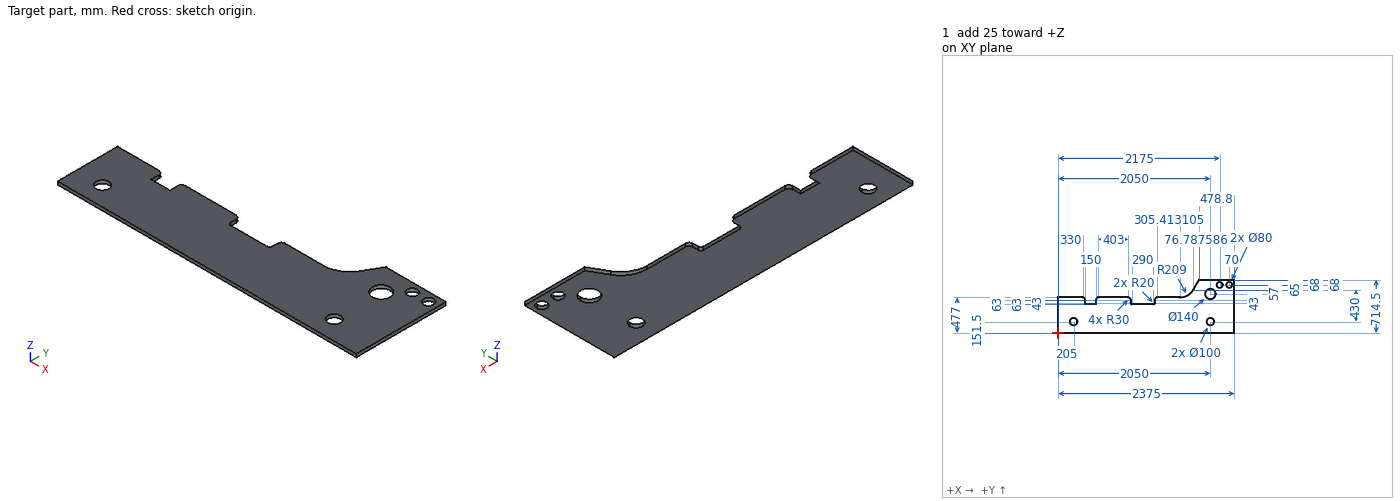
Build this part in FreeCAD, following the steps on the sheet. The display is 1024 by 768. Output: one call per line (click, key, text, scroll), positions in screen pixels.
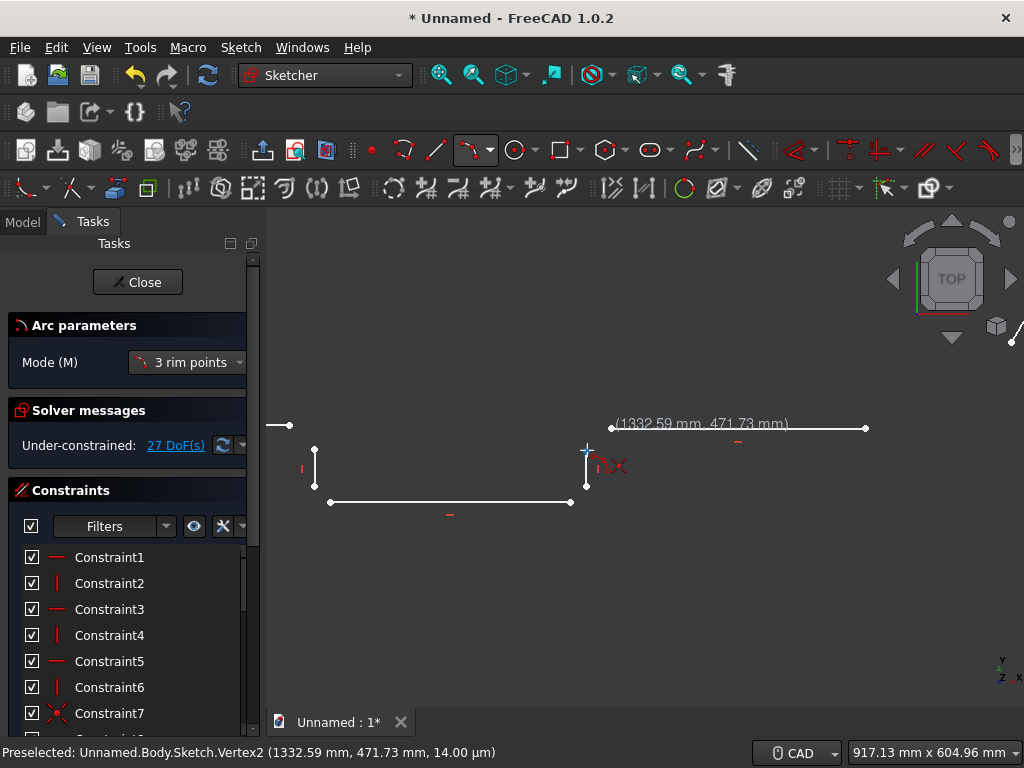
click(586, 452)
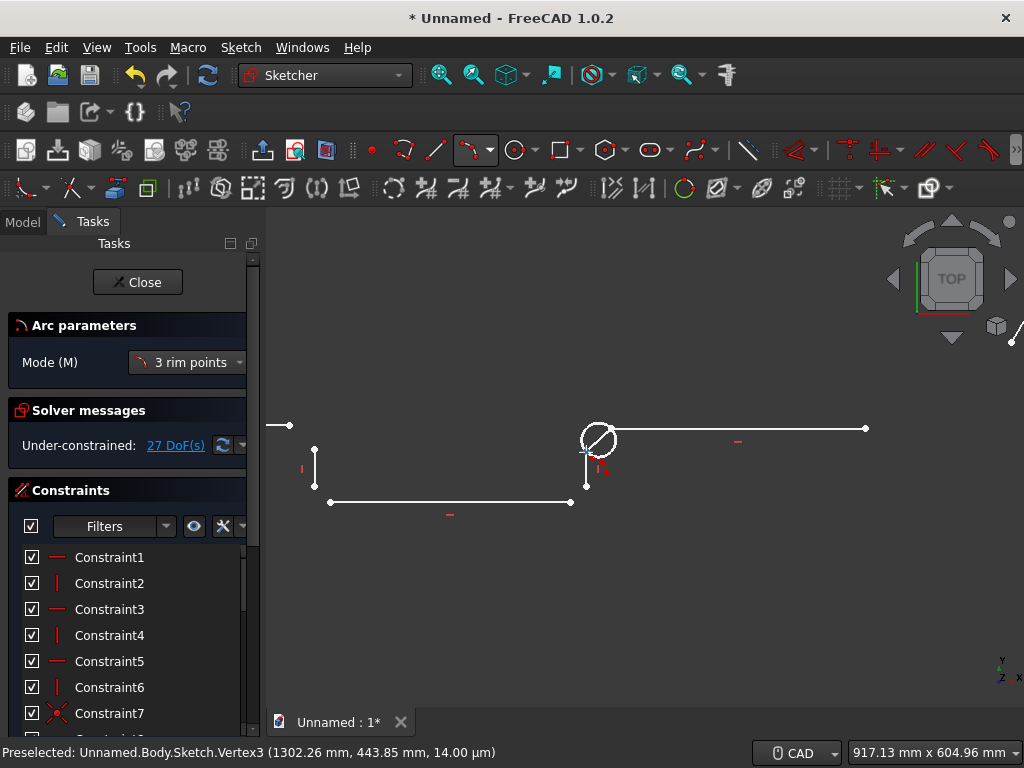
scroll(594, 431, up, 4)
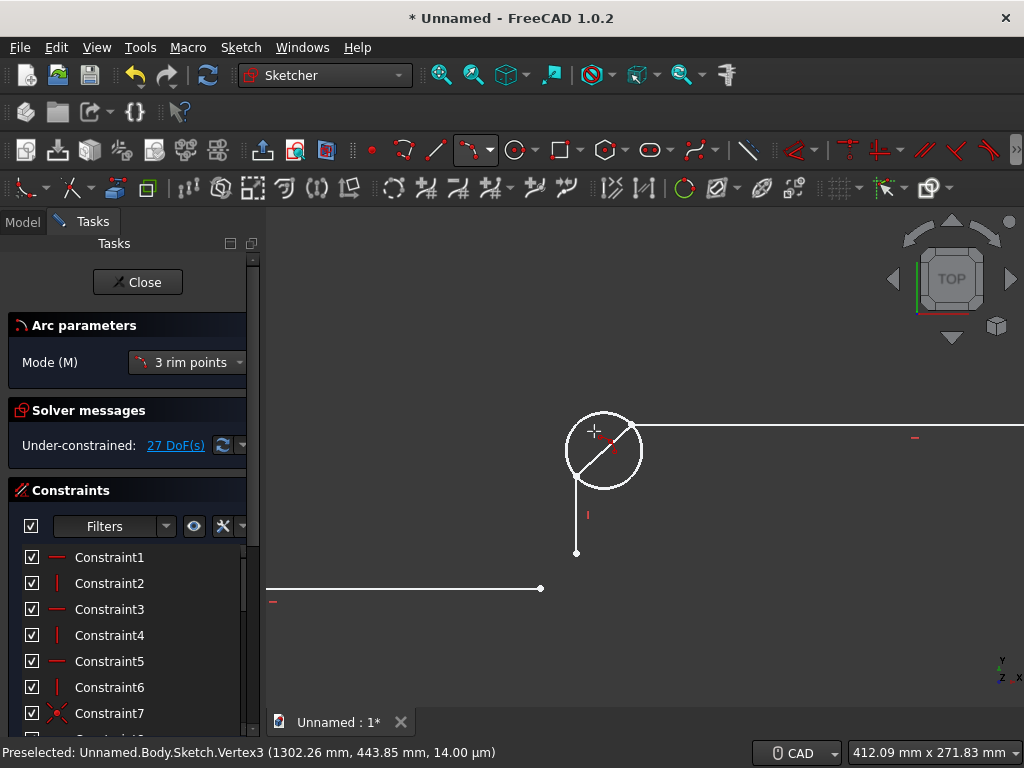
click(594, 431)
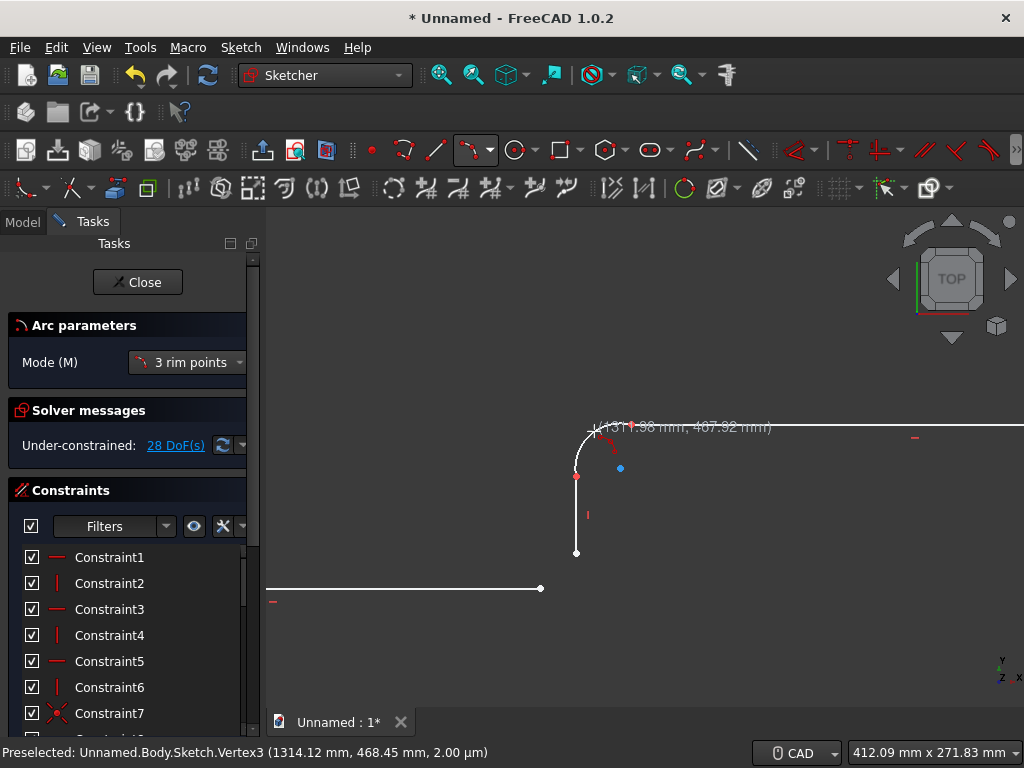
click(576, 553)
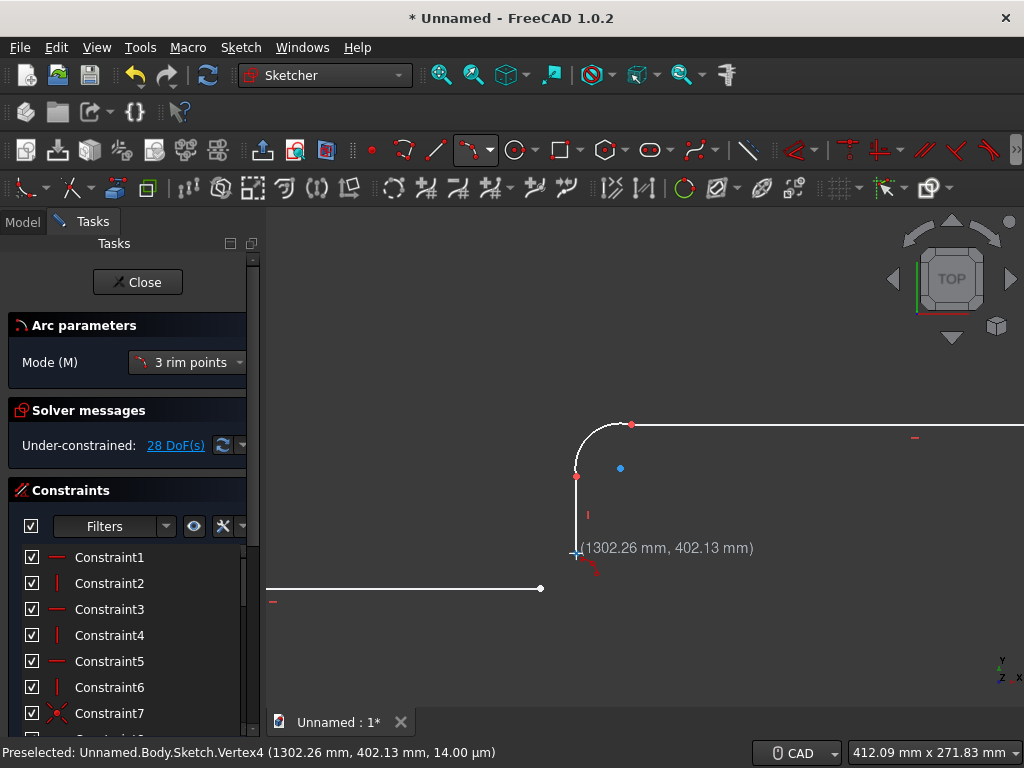
scroll(598, 439, down, 12)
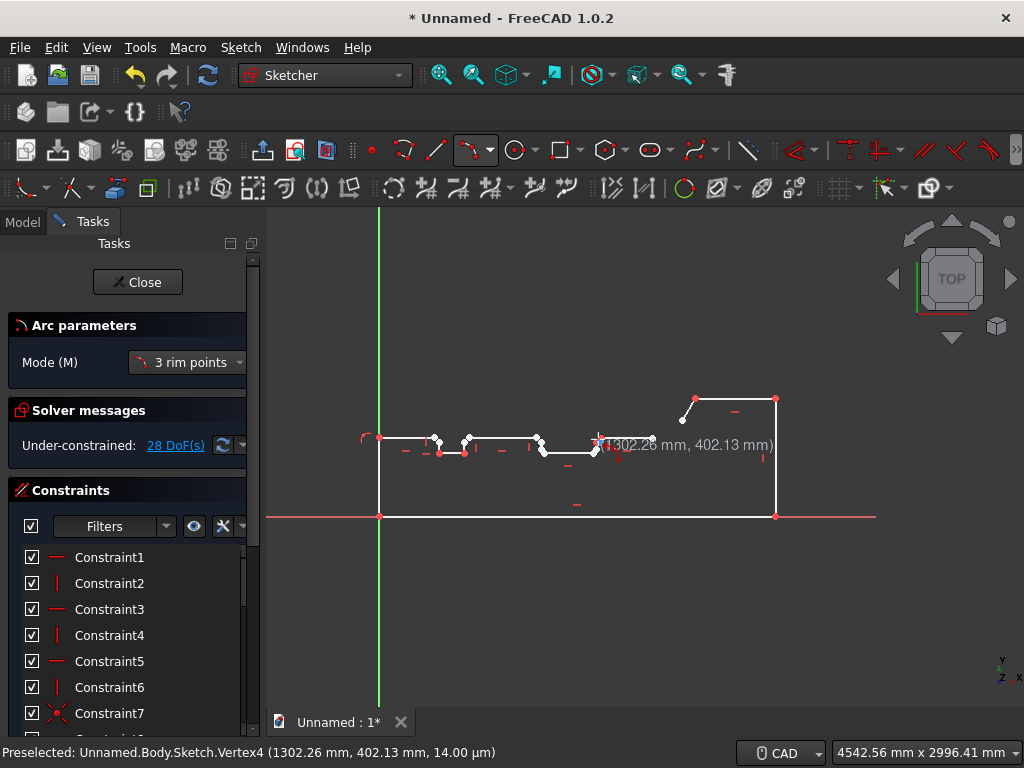
scroll(593, 453, up, 7)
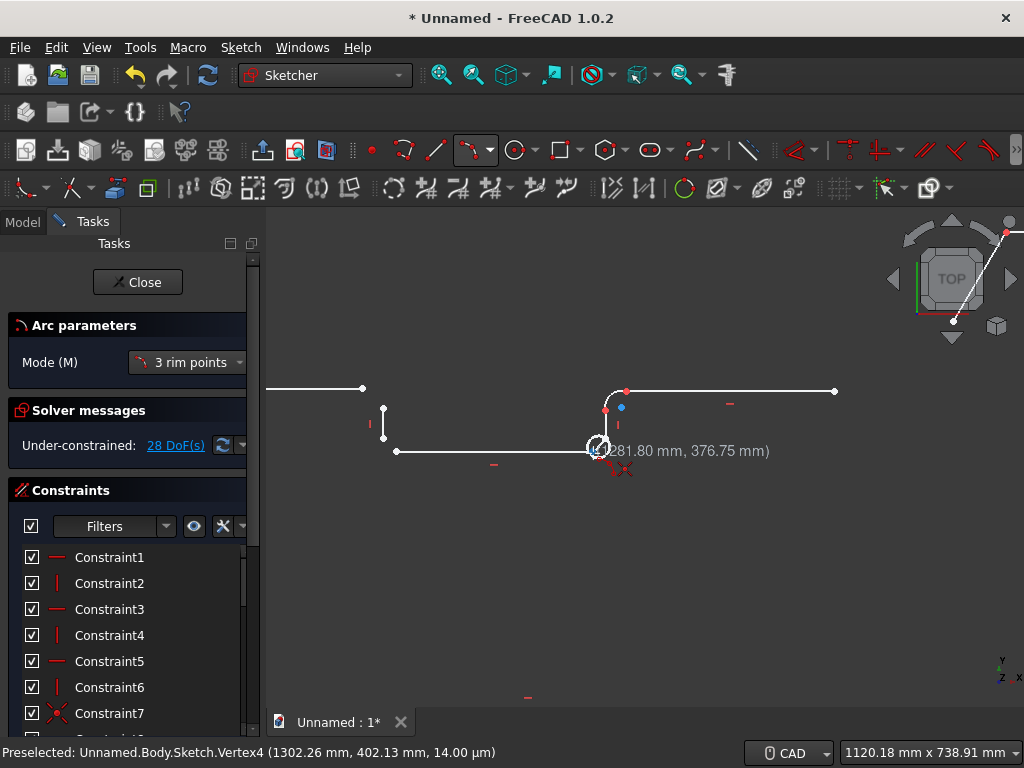
click(592, 452)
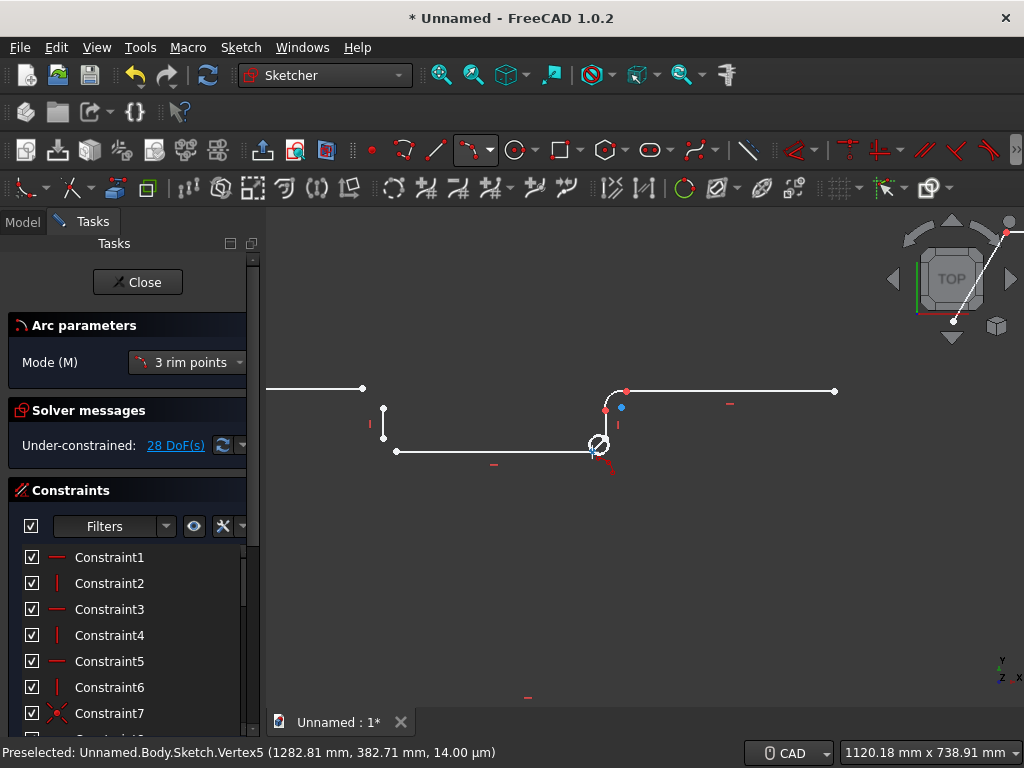
scroll(602, 447, up, 7)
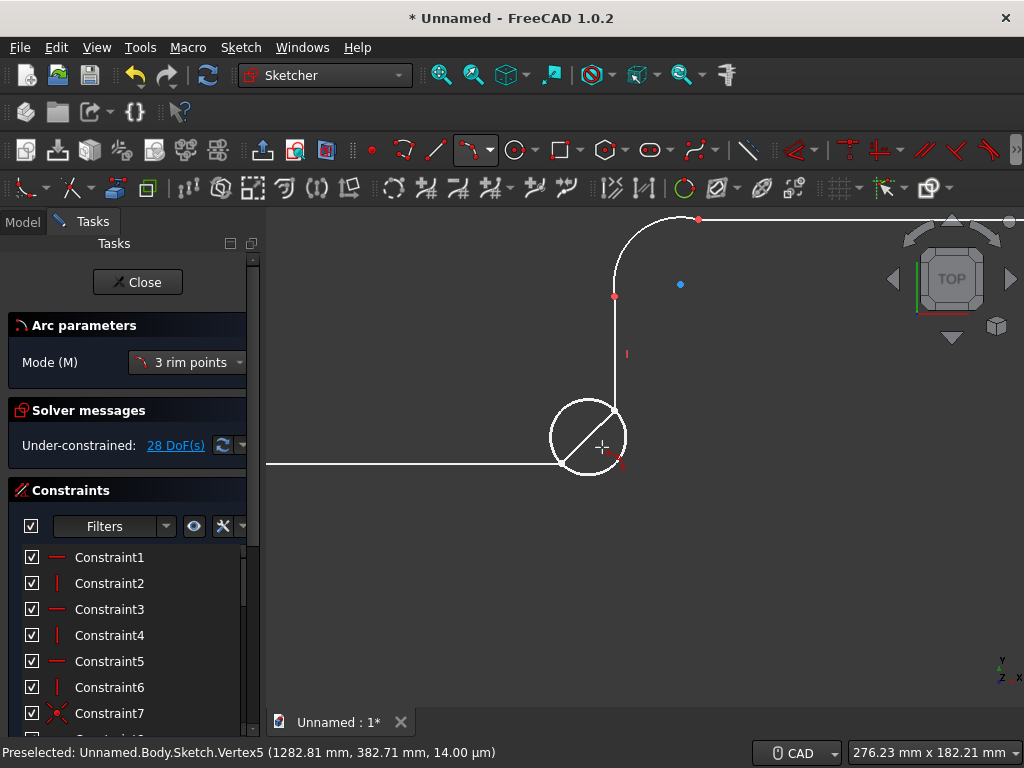
click(601, 444)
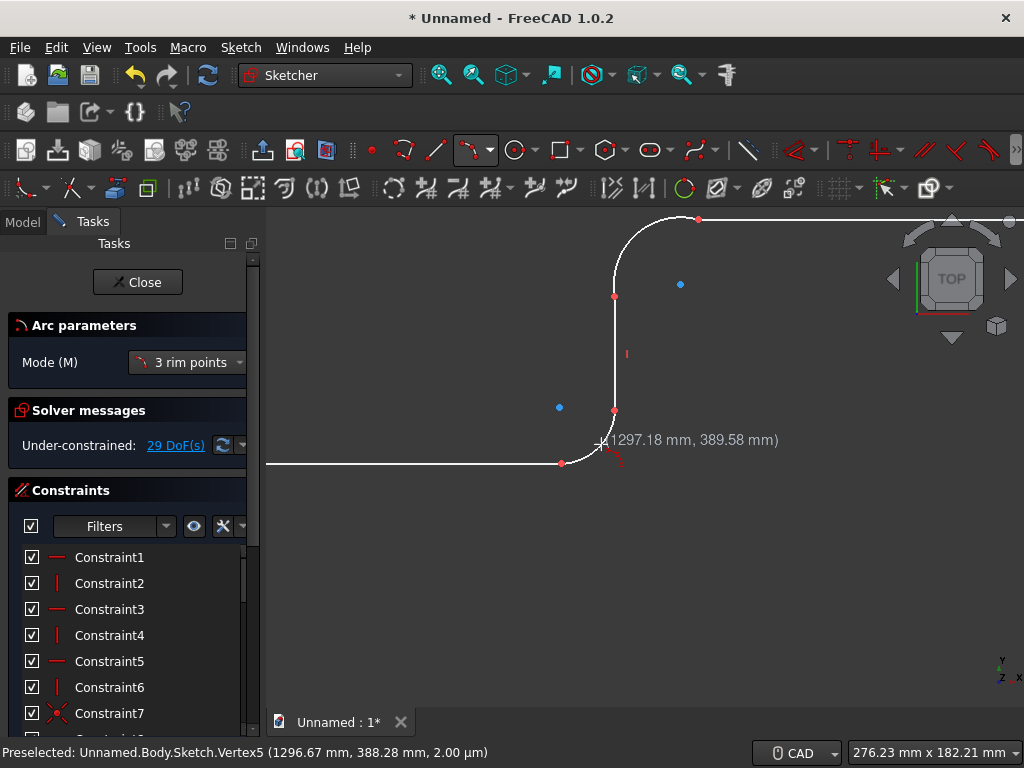
scroll(594, 452, down, 14)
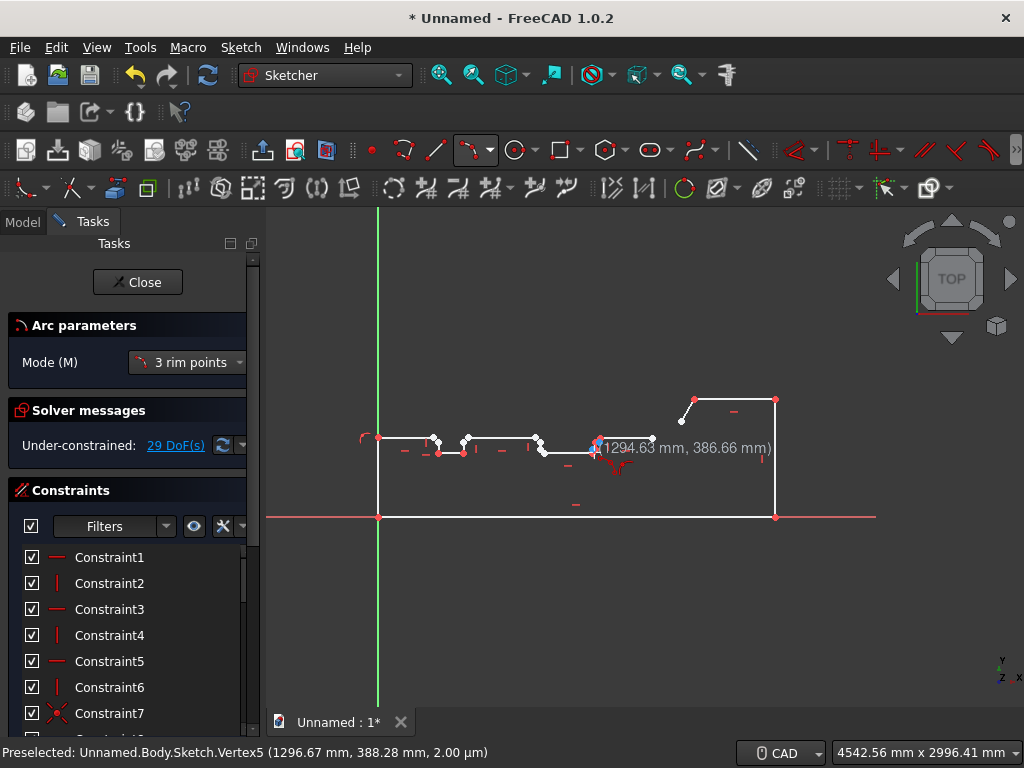
scroll(544, 453, up, 7)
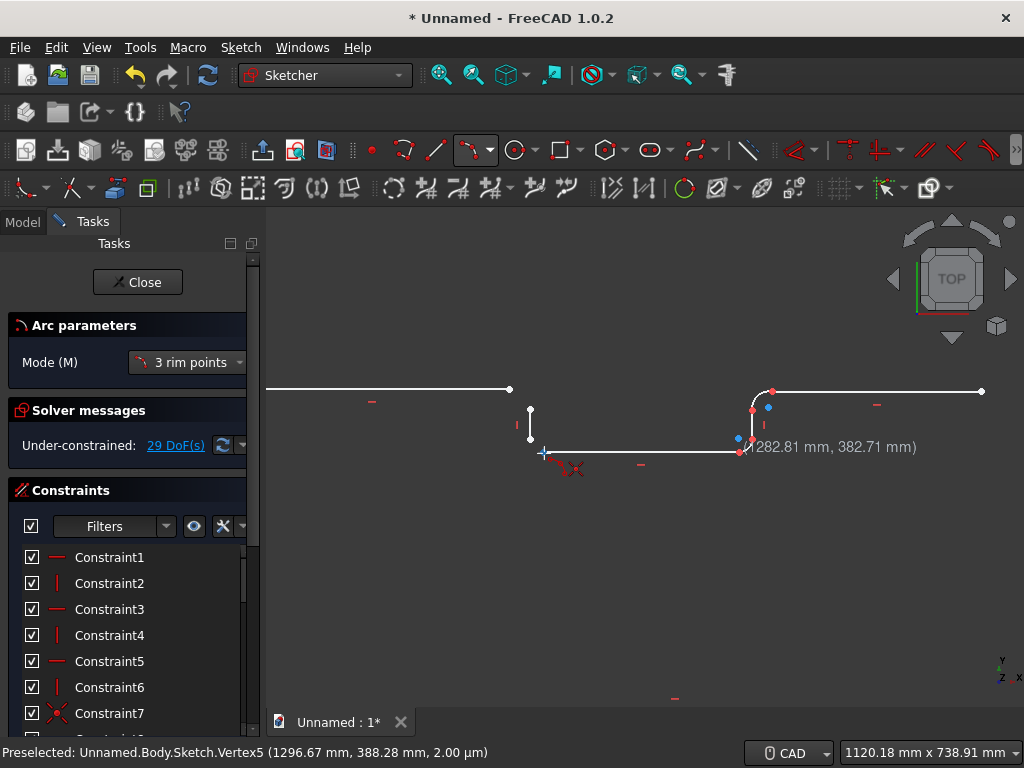
click(543, 452)
click(530, 439)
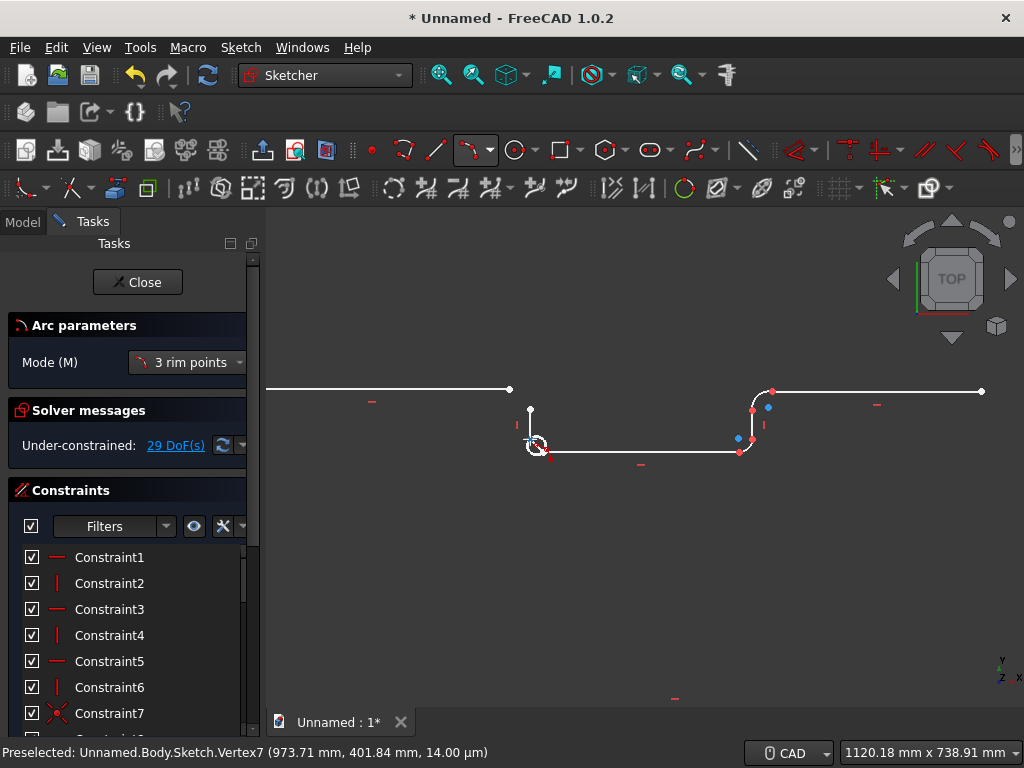
scroll(534, 447, up, 7)